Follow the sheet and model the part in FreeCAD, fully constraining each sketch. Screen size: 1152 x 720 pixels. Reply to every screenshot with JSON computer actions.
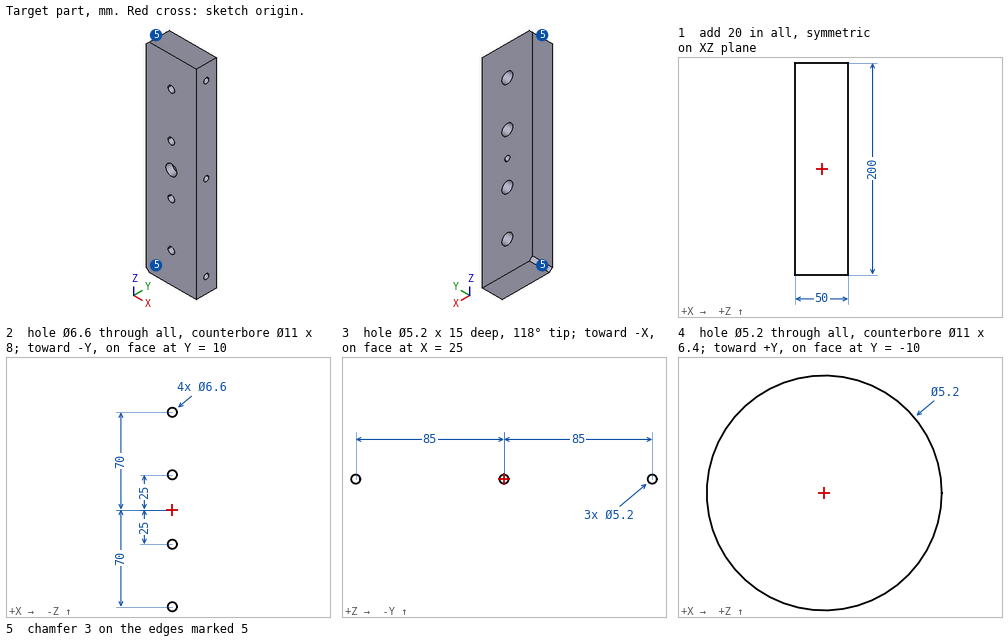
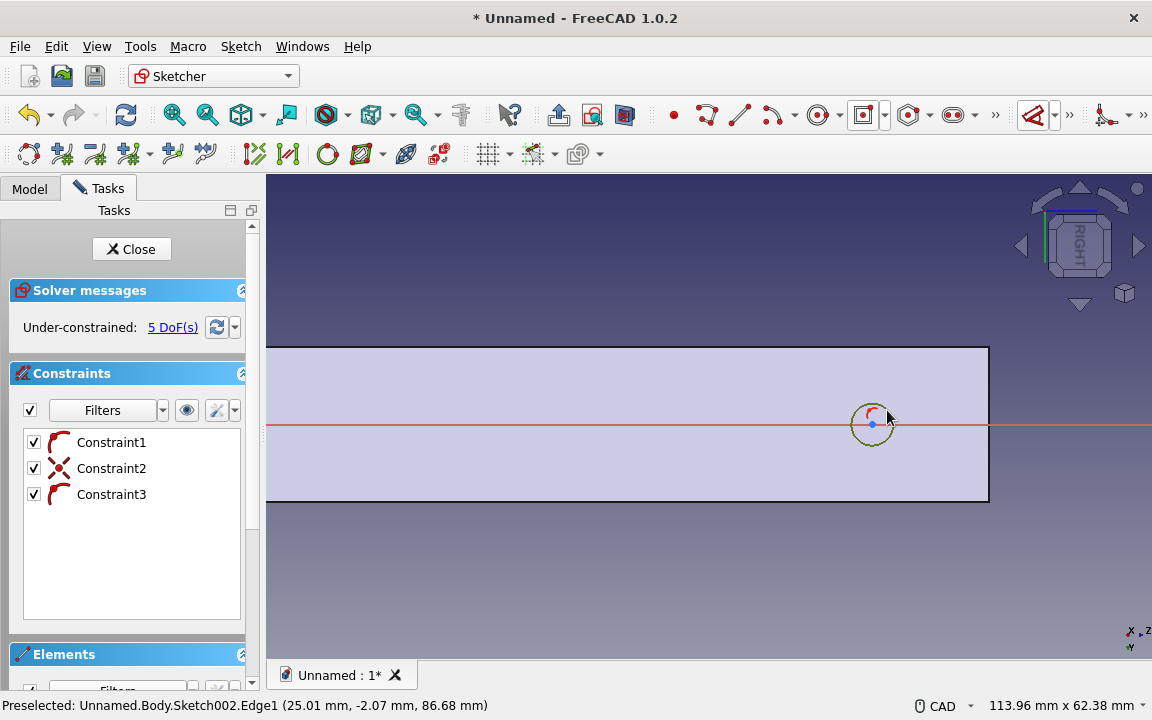
{"action": "scroll", "coordinate": [890, 412], "scroll_direction": "down", "scroll_amount": 5}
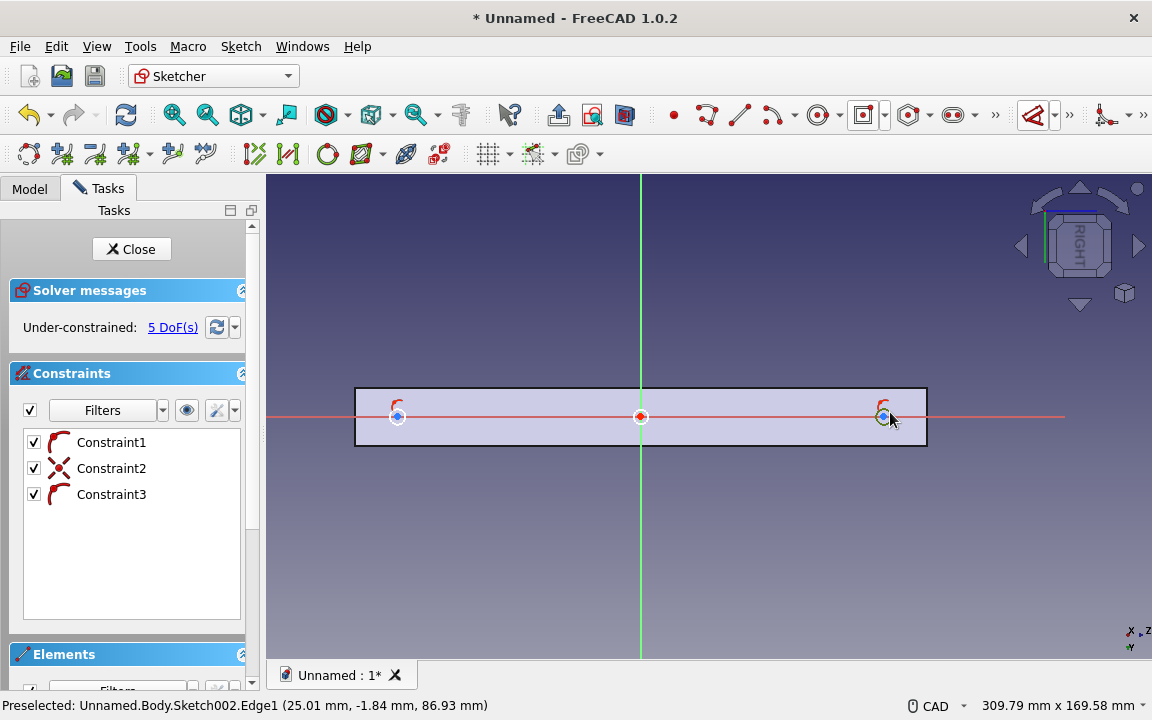
{"action": "scroll", "coordinate": [646, 412], "scroll_direction": "up", "scroll_amount": 5}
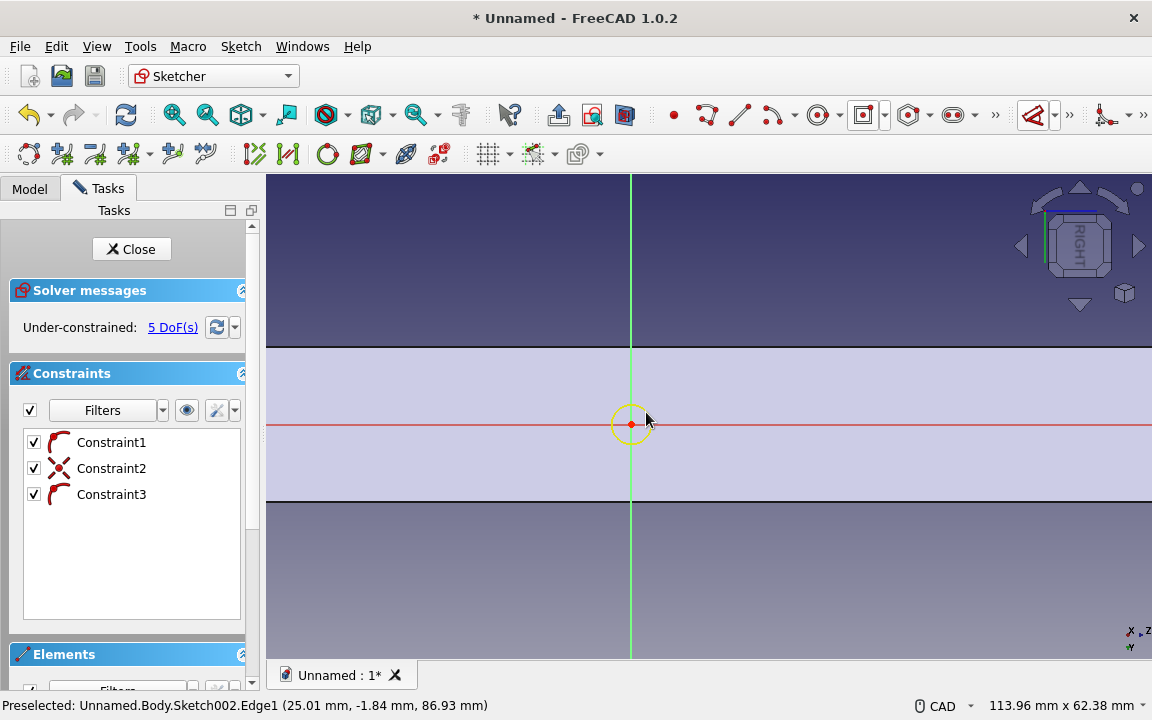
{"action": "left_click", "coordinate": [645, 411]}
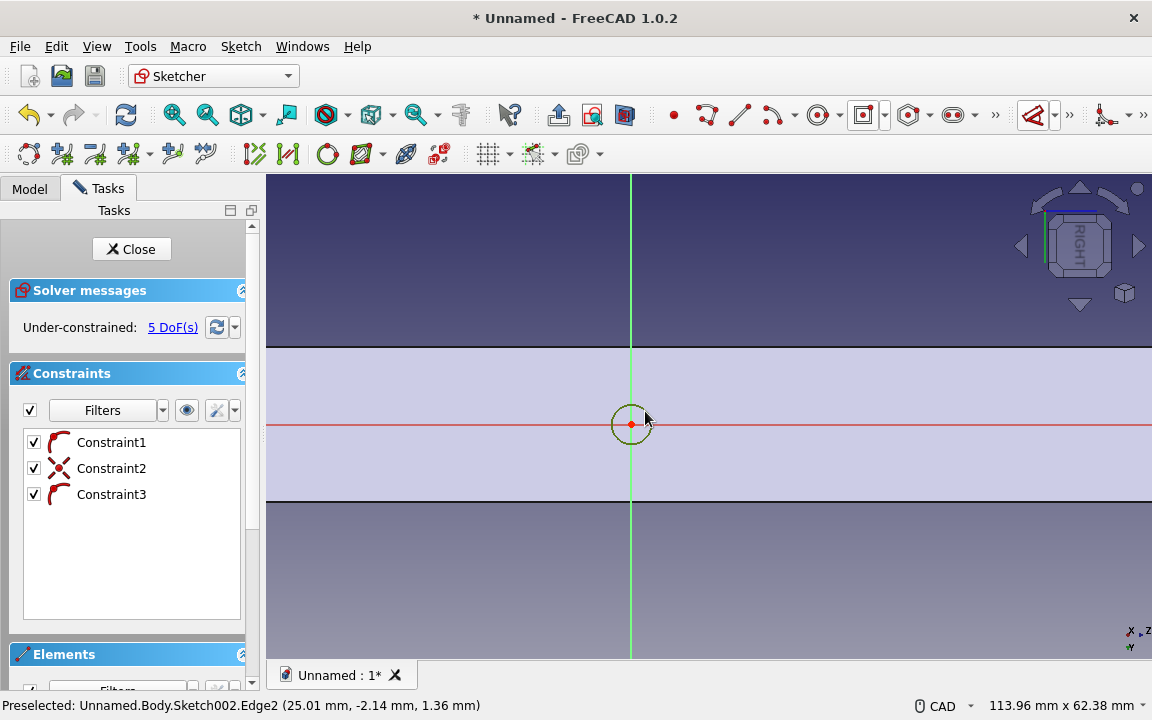
{"action": "scroll", "coordinate": [646, 412], "scroll_direction": "down", "scroll_amount": 5}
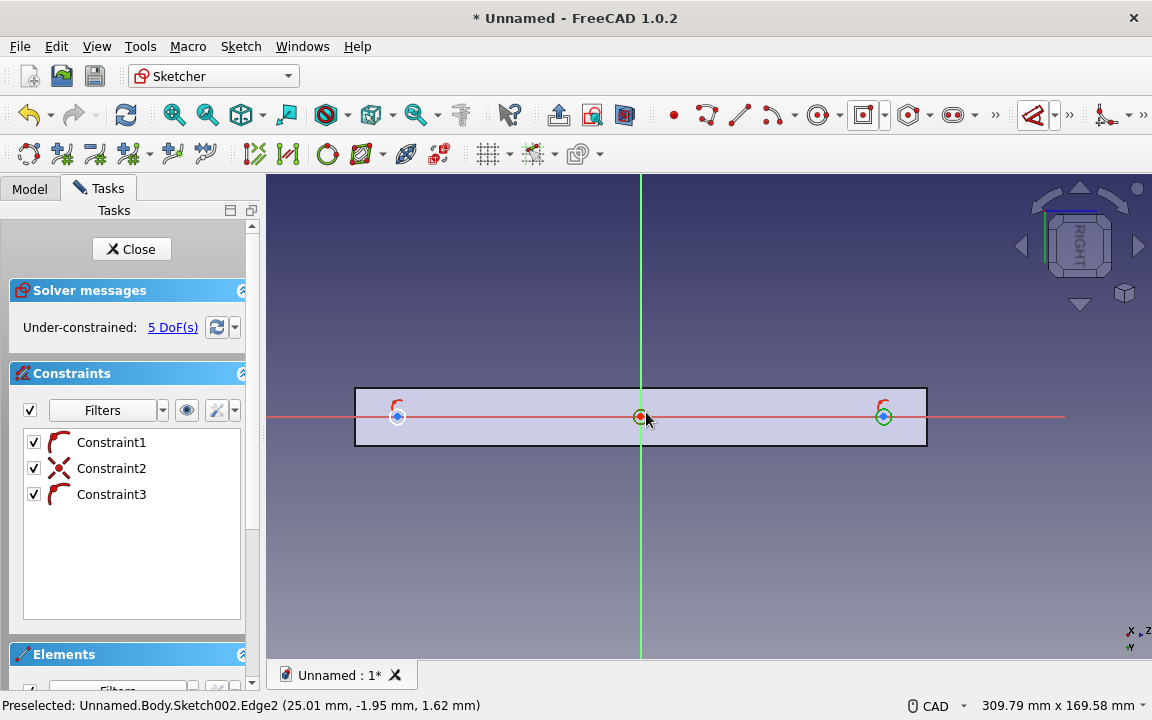
{"action": "scroll", "coordinate": [403, 412], "scroll_direction": "up", "scroll_amount": 5}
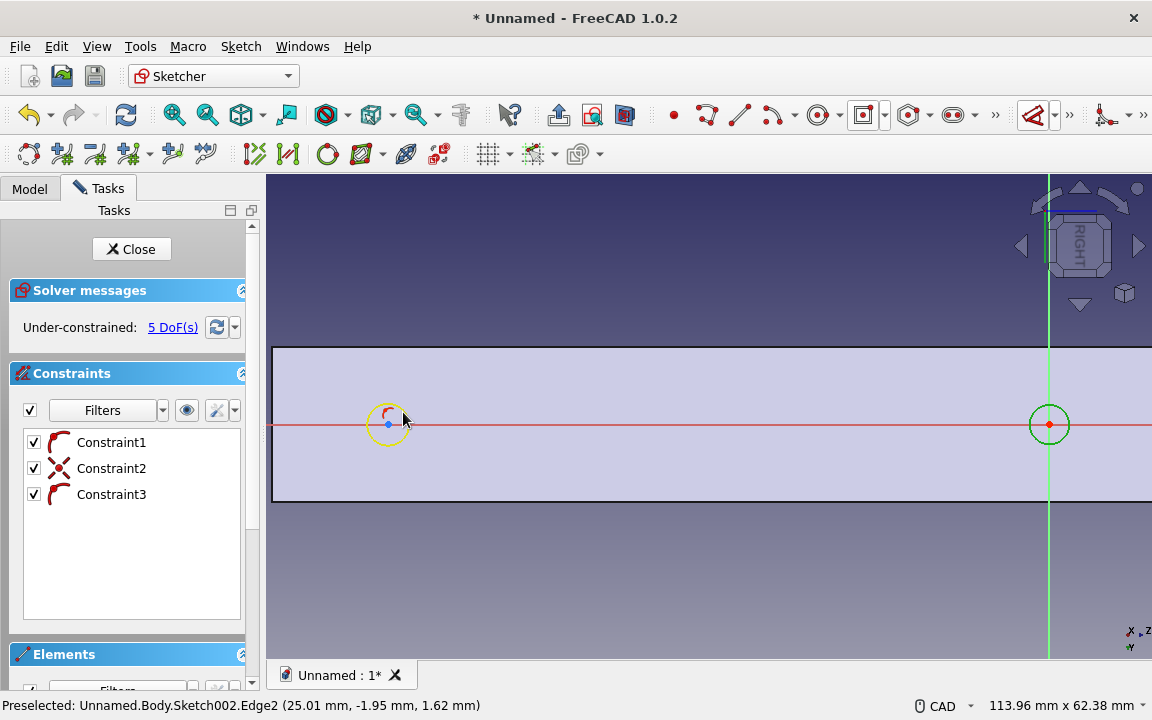
{"action": "left_click", "coordinate": [403, 410]}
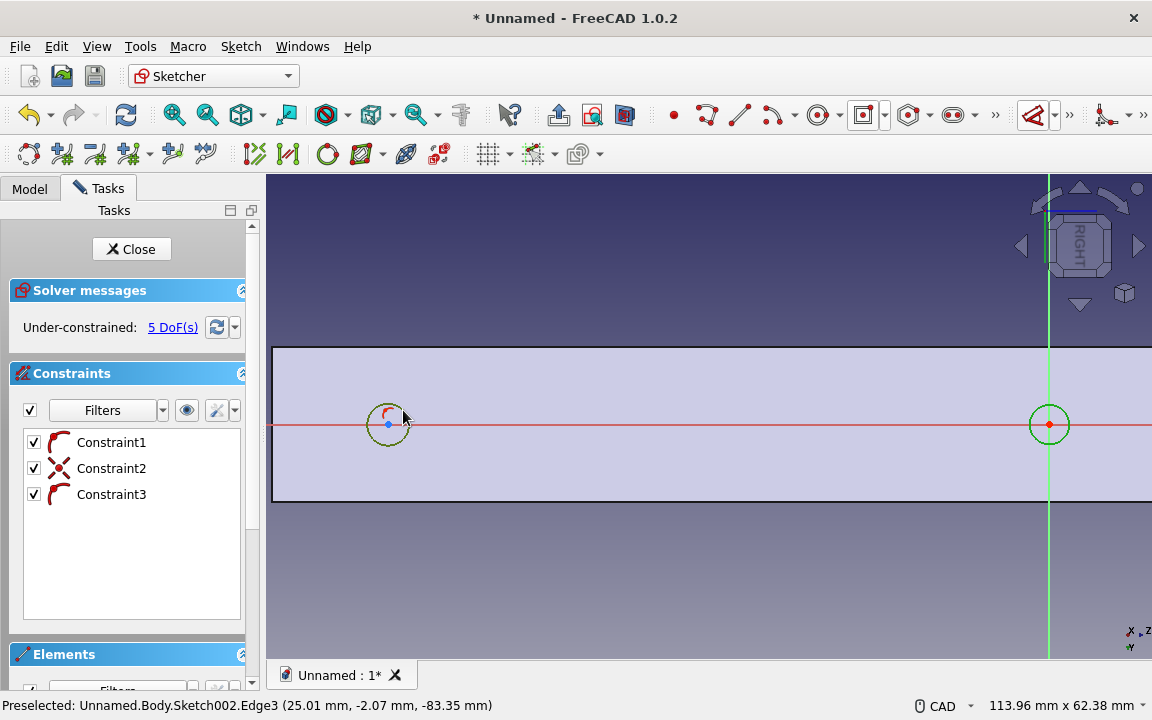
{"action": "key", "text": "e"}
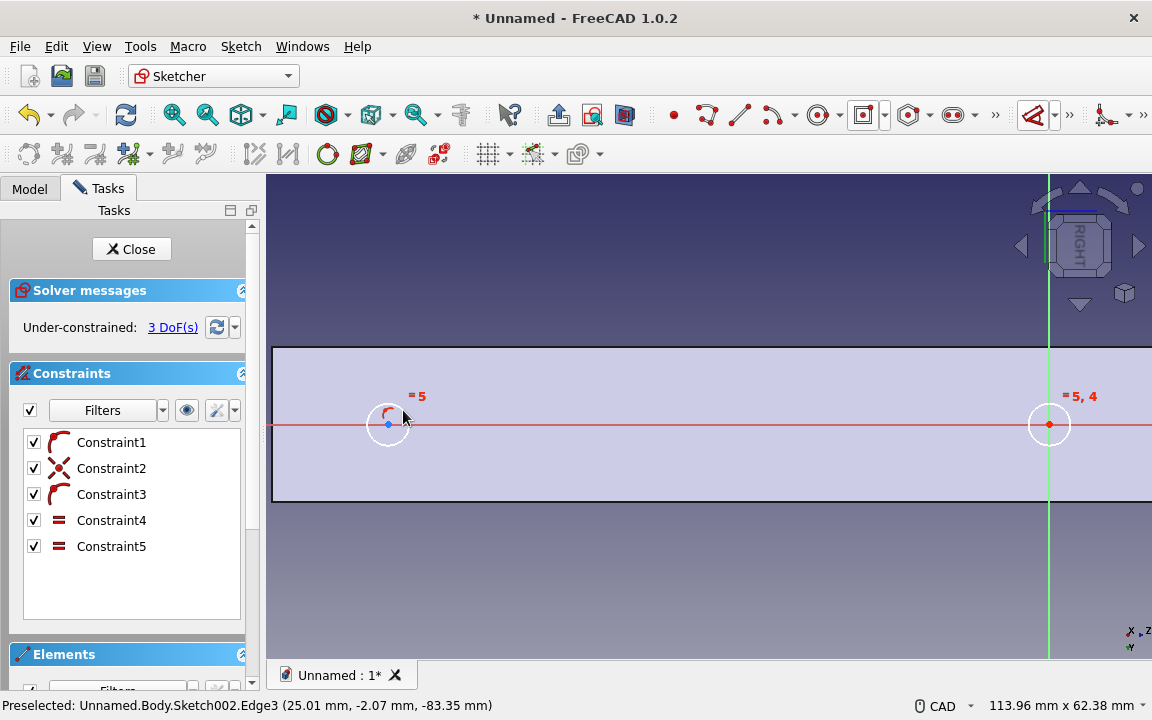
{"action": "scroll", "coordinate": [402, 412], "scroll_direction": "down", "scroll_amount": 5}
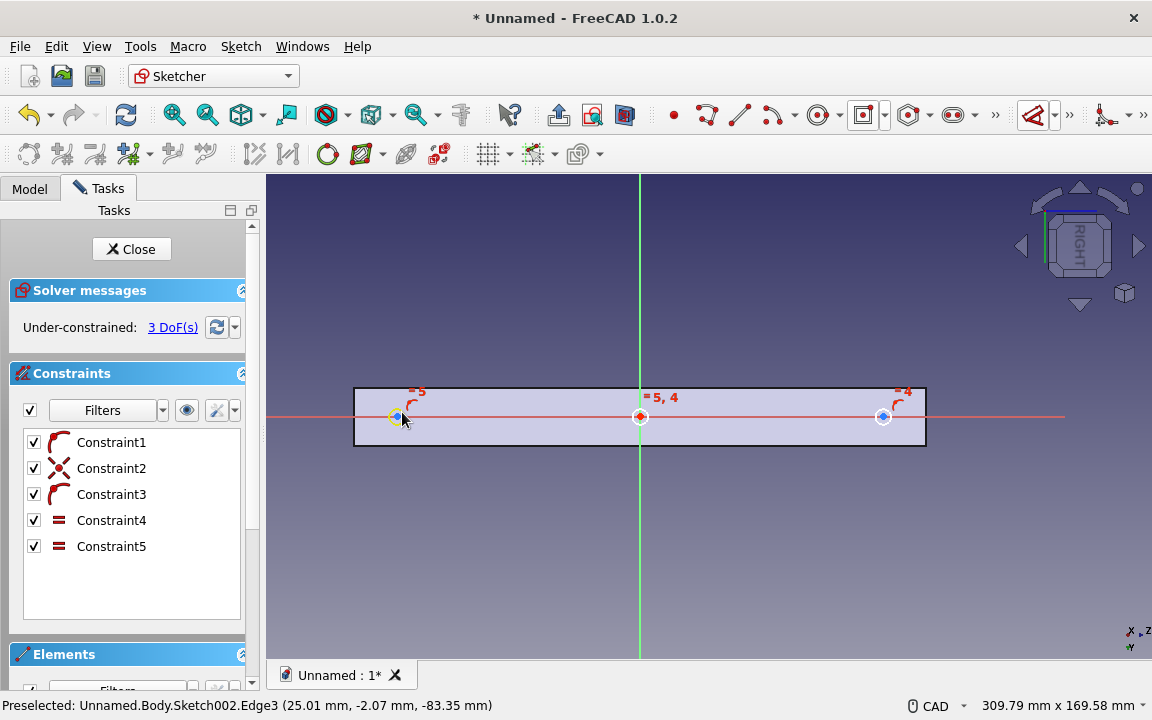
{"action": "scroll", "coordinate": [889, 412], "scroll_direction": "up", "scroll_amount": 5}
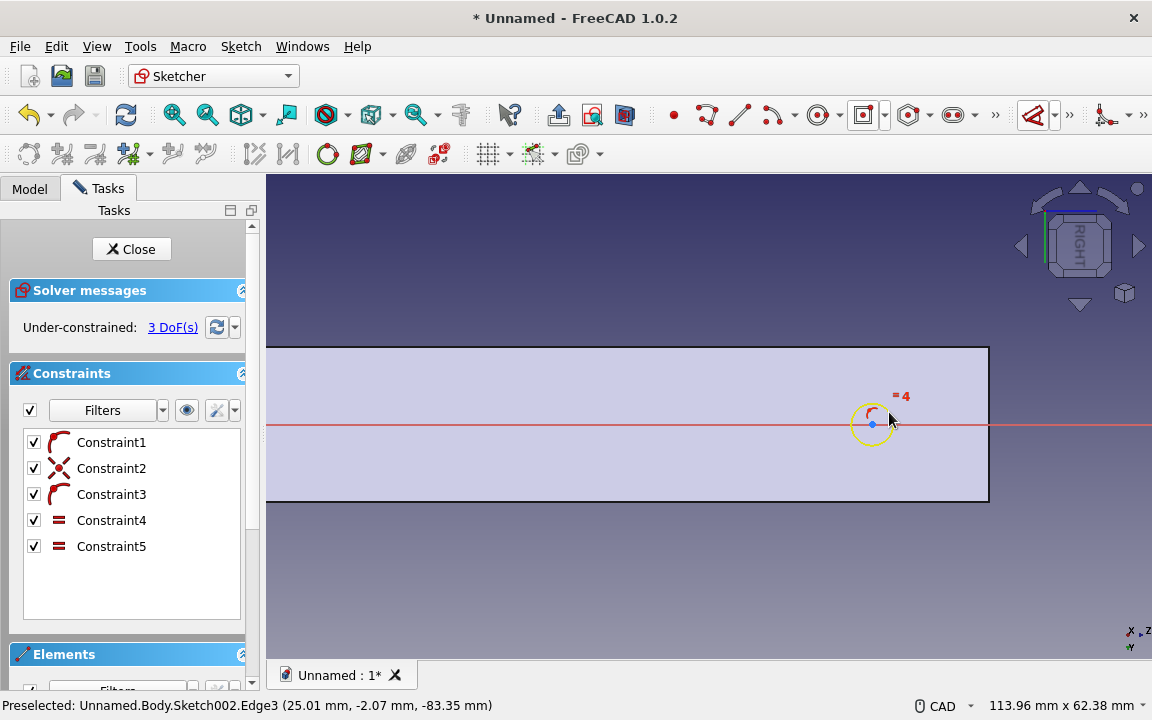
{"action": "left_click", "coordinate": [887, 410]}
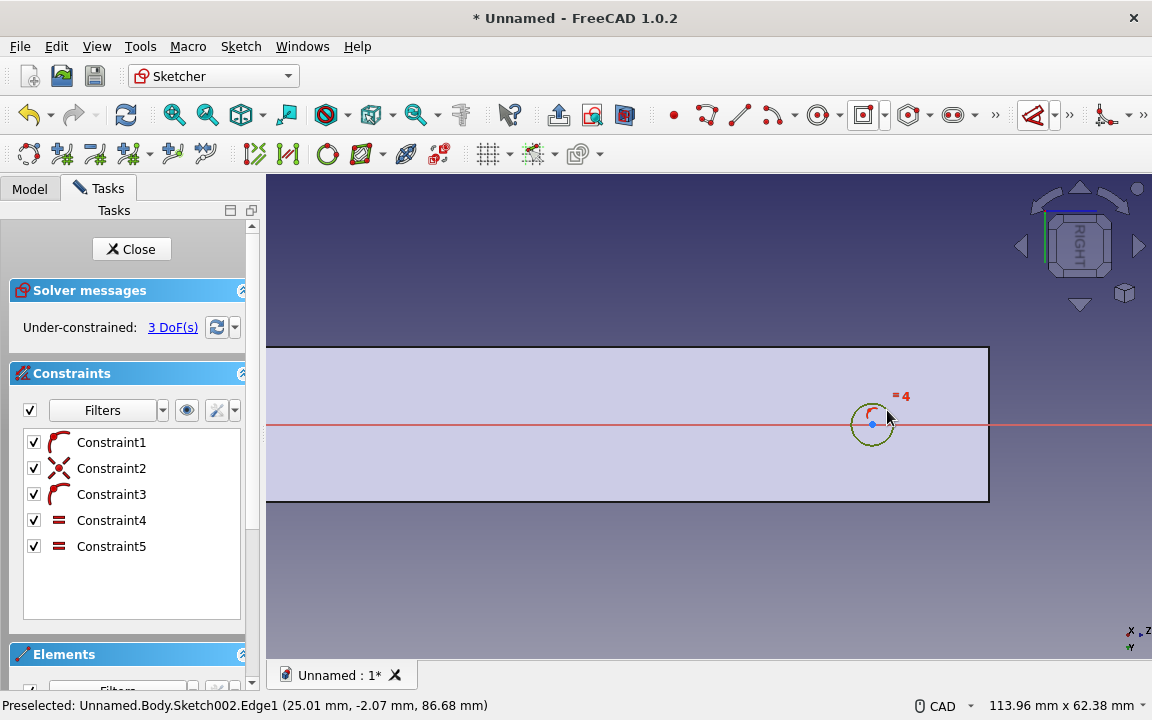
{"action": "left_click", "coordinate": [1054, 116]}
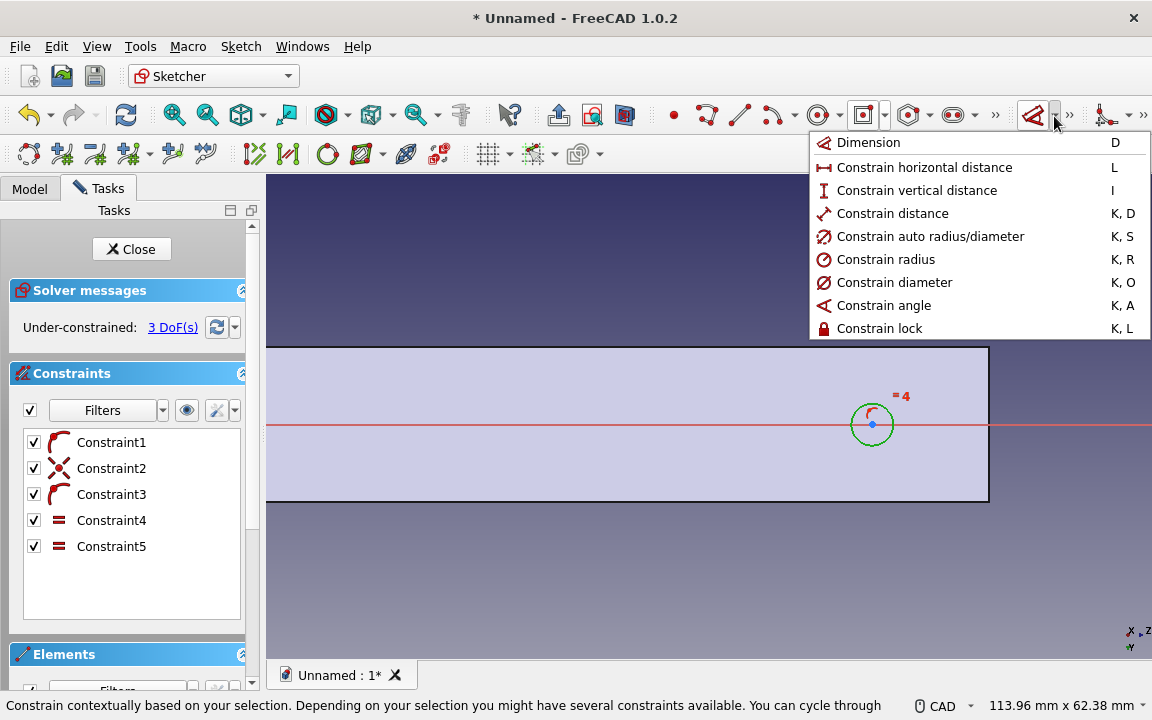
{"action": "left_click", "coordinate": [980, 282]}